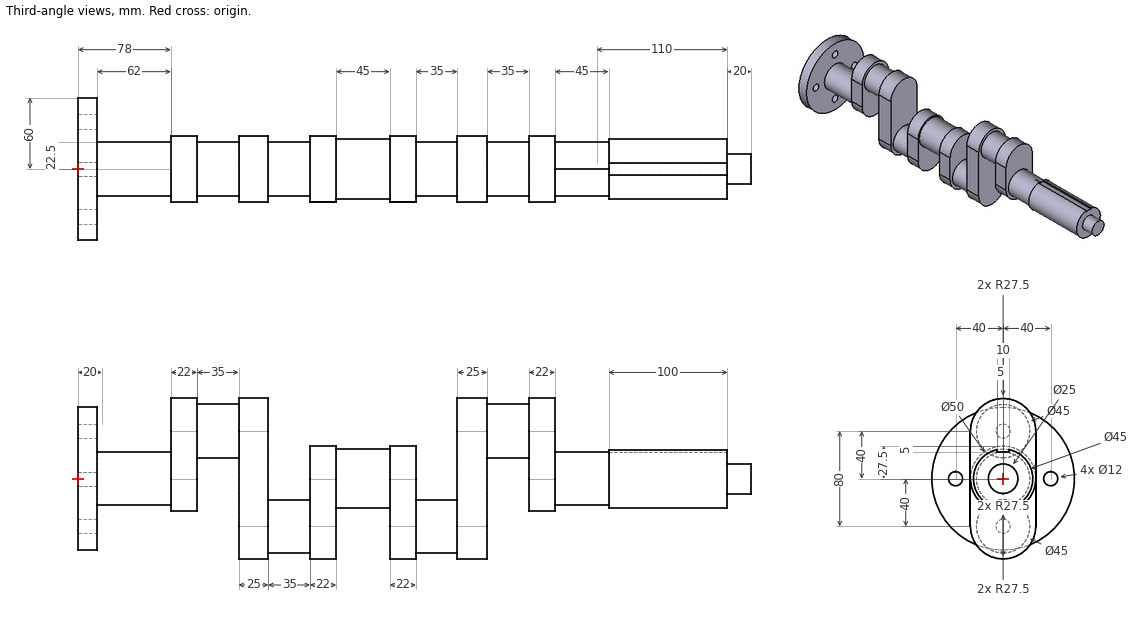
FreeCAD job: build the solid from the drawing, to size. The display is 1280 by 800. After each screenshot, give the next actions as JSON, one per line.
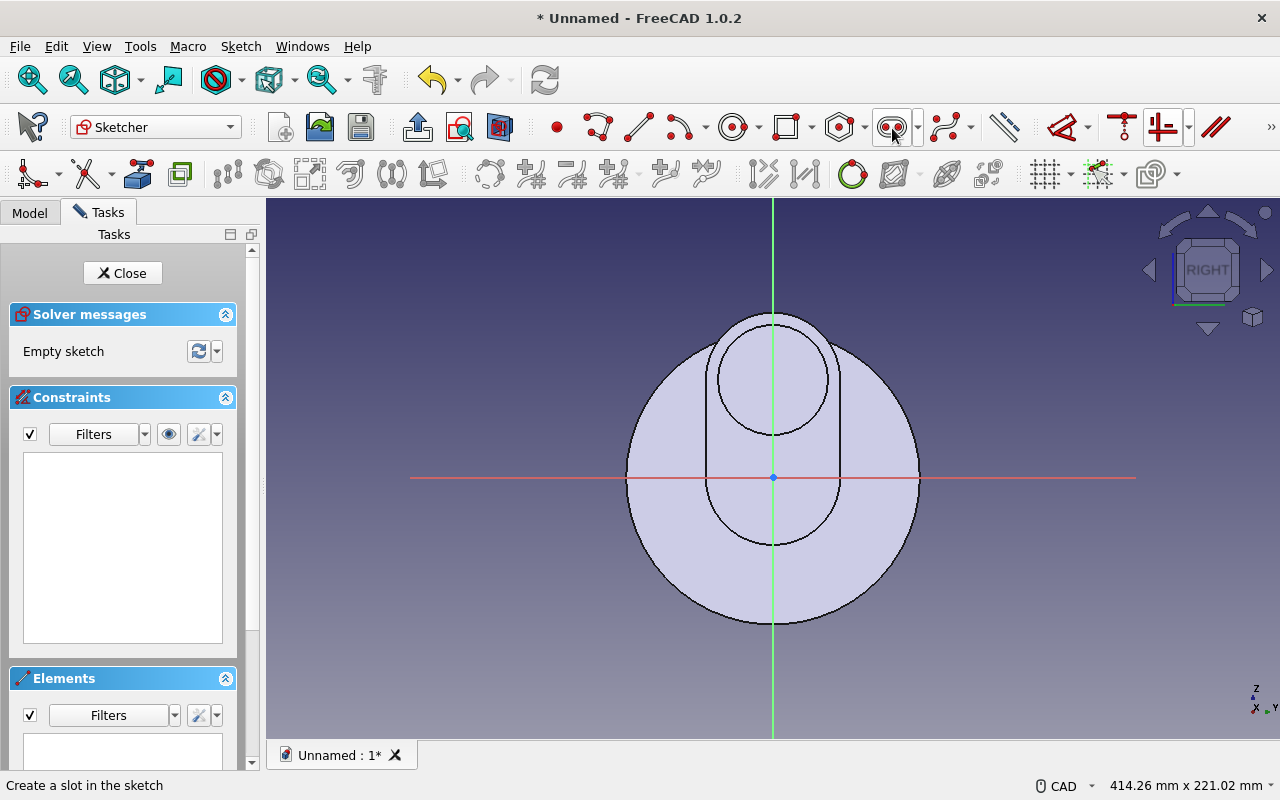
{"action": "left_click", "coordinate": [773, 576]}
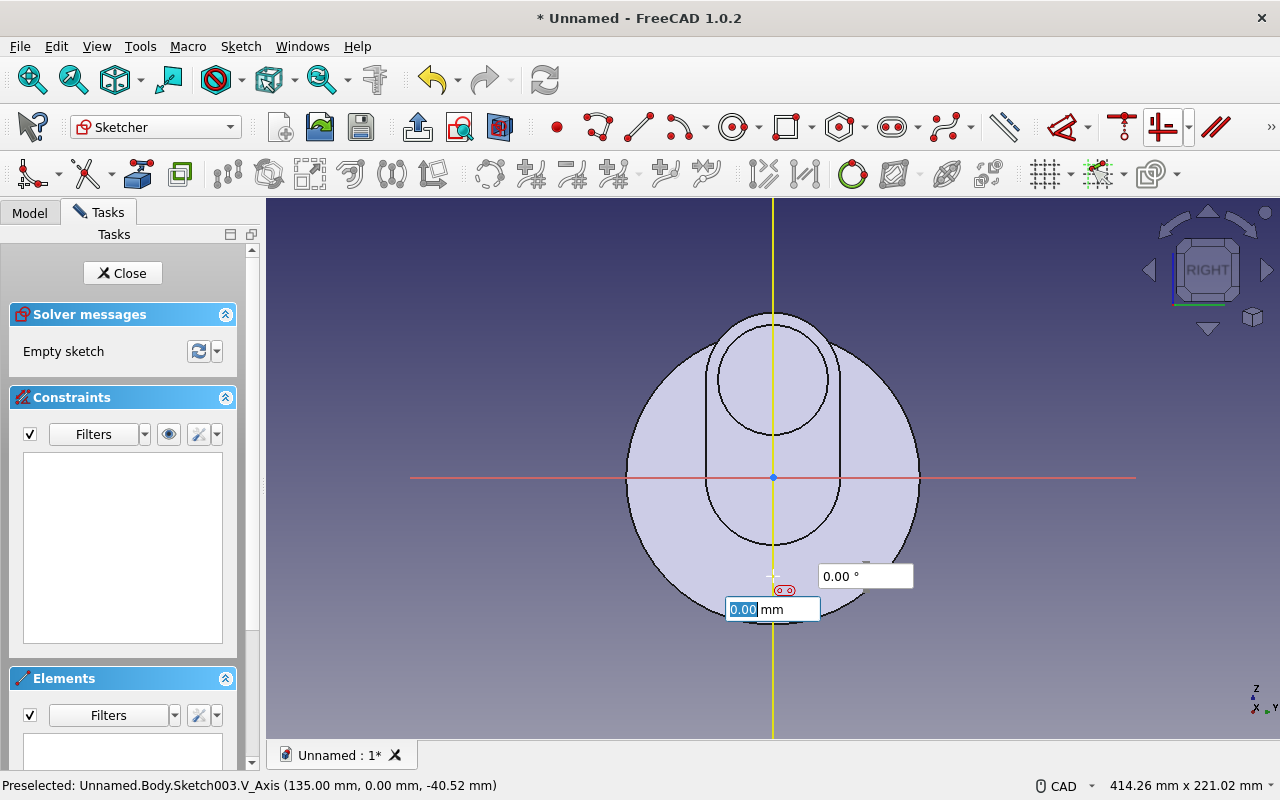
{"action": "left_click", "coordinate": [782, 380]}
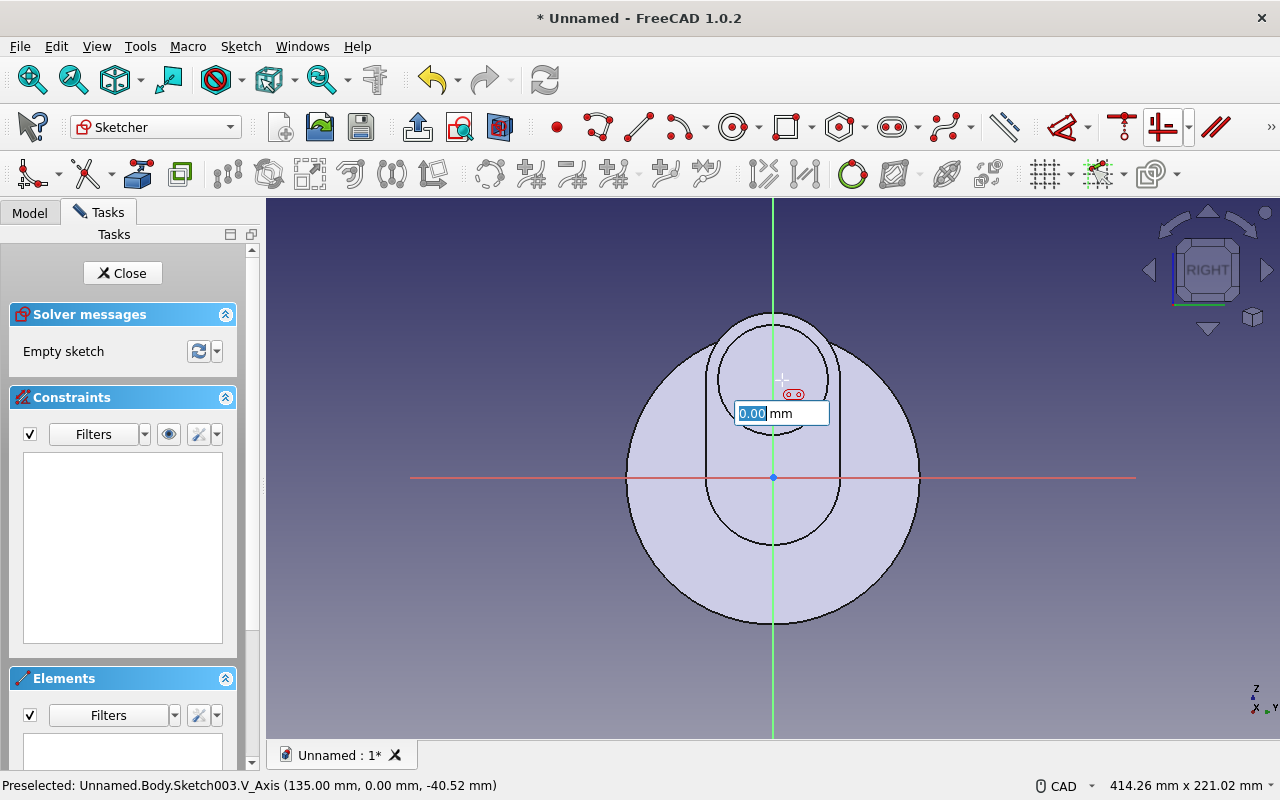
{"action": "left_click", "coordinate": [840, 507]}
{"action": "key", "text": "Escape"}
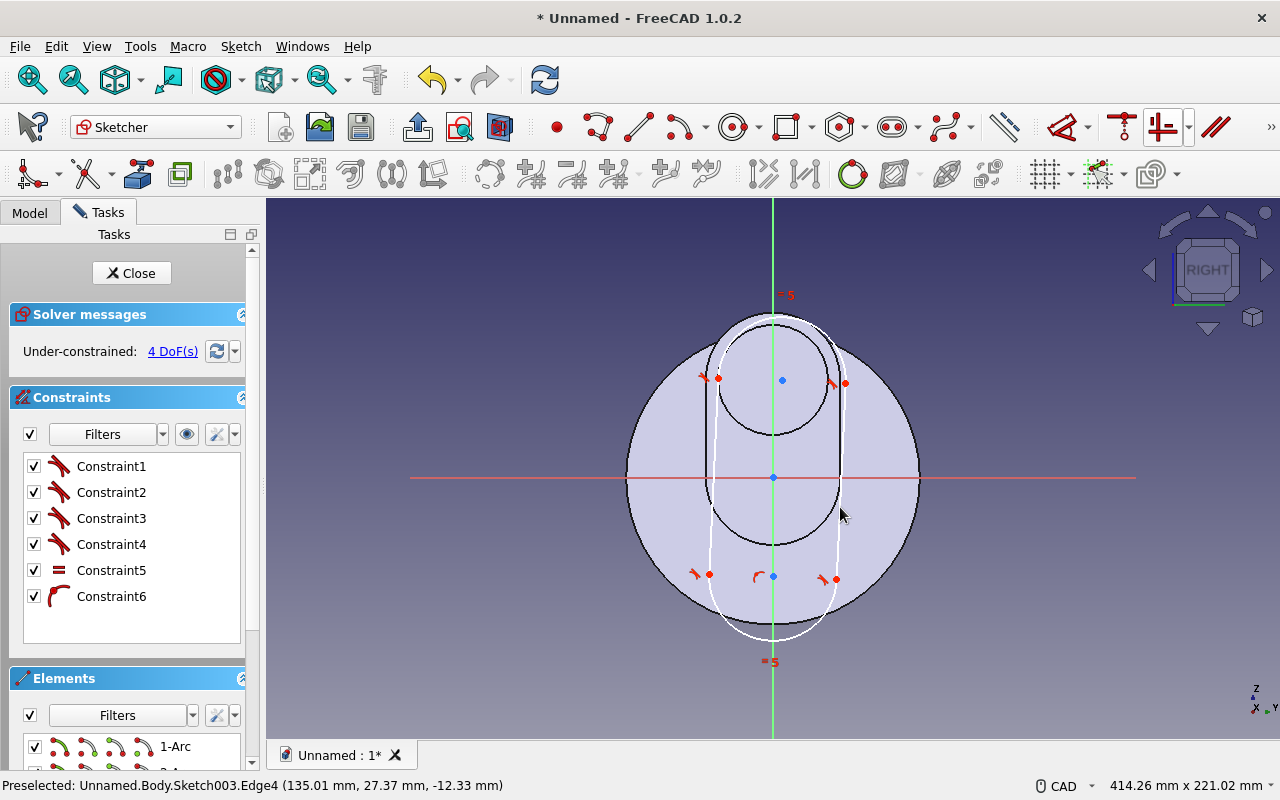
{"action": "left_click", "coordinate": [712, 515]}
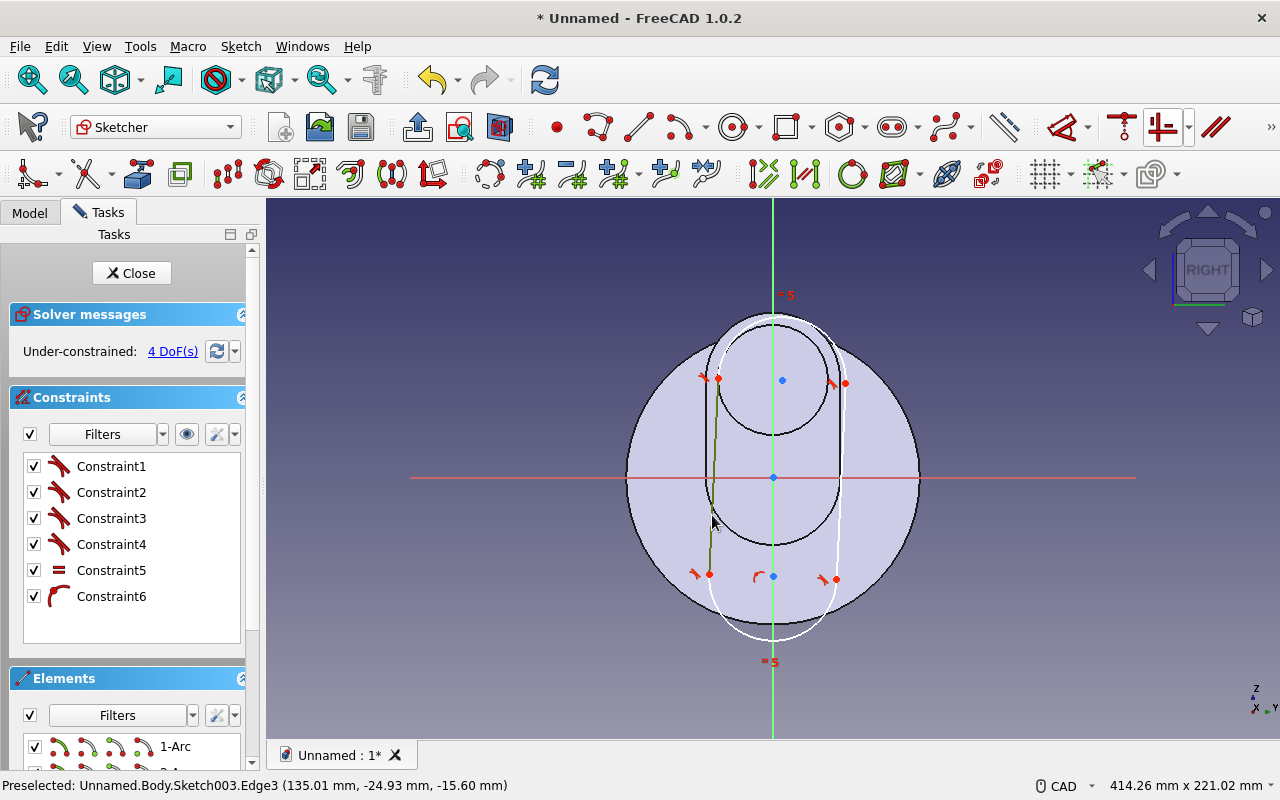
{"action": "left_click", "coordinate": [1188, 128]}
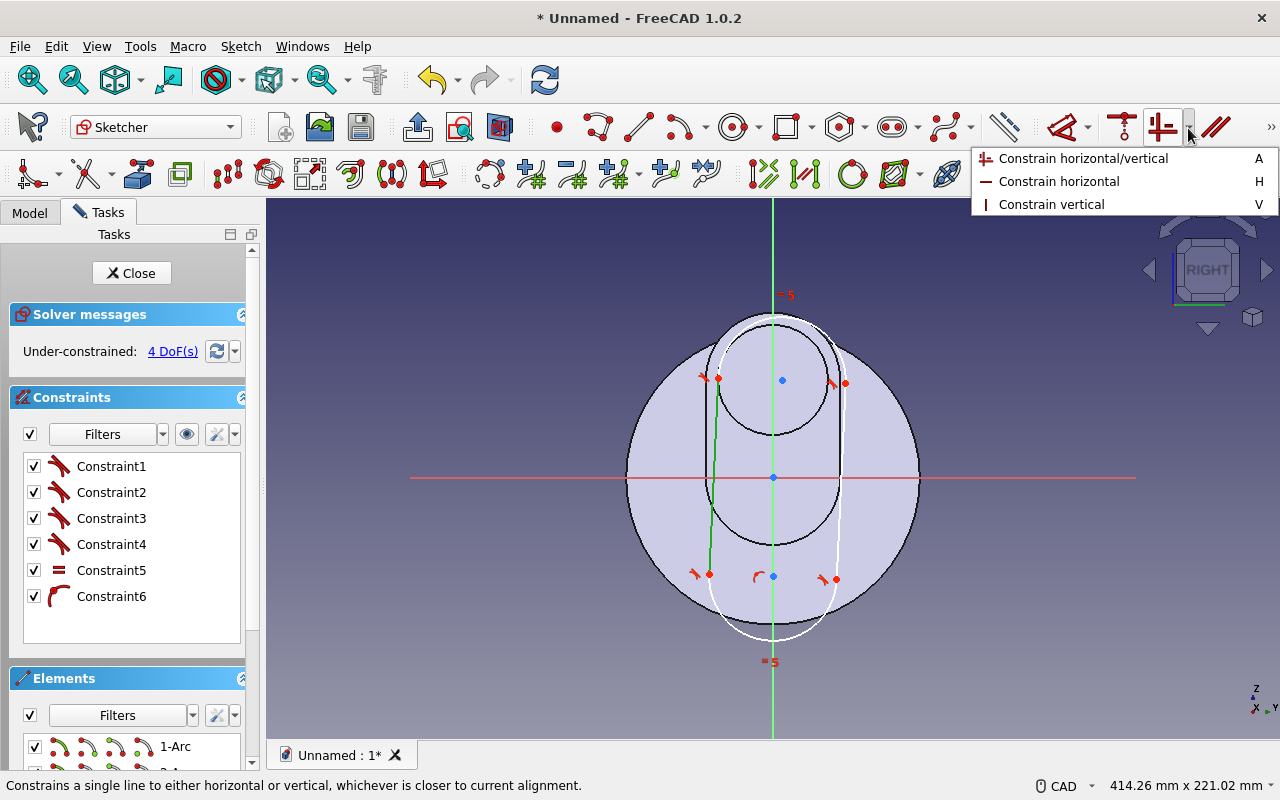
{"action": "left_click", "coordinate": [1125, 204]}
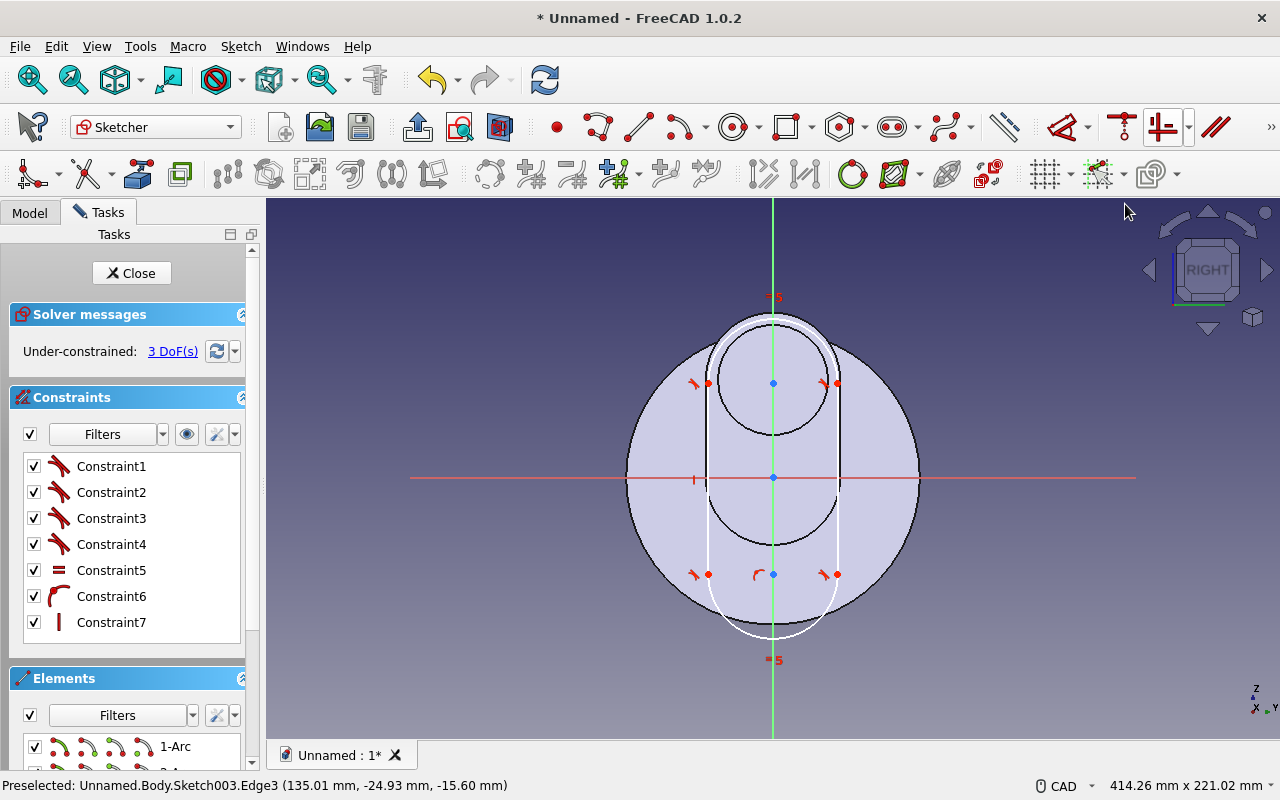
{"action": "left_click", "coordinate": [1062, 128]}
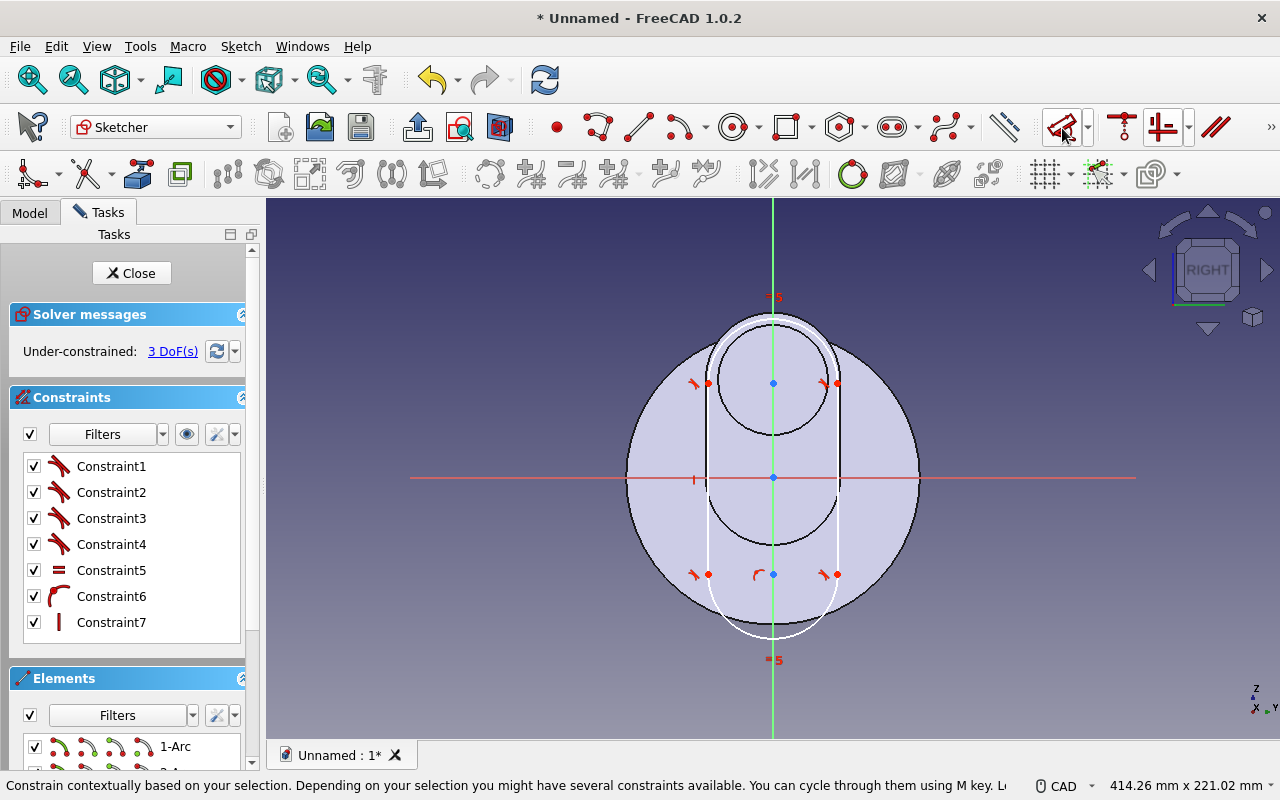
{"action": "left_click", "coordinate": [735, 626]}
{"action": "left_click", "coordinate": [716, 652]}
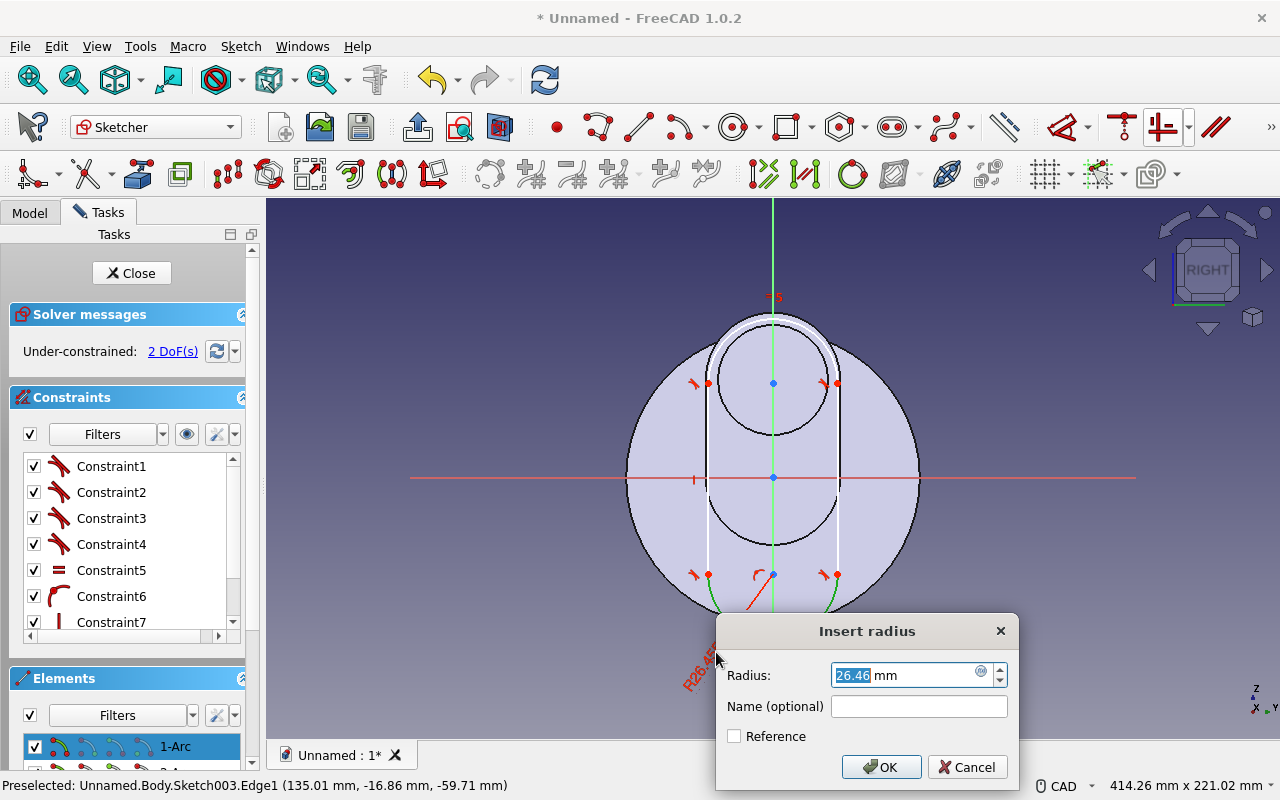
{"action": "type", "text": "27.5"}
{"action": "key", "text": "Return"}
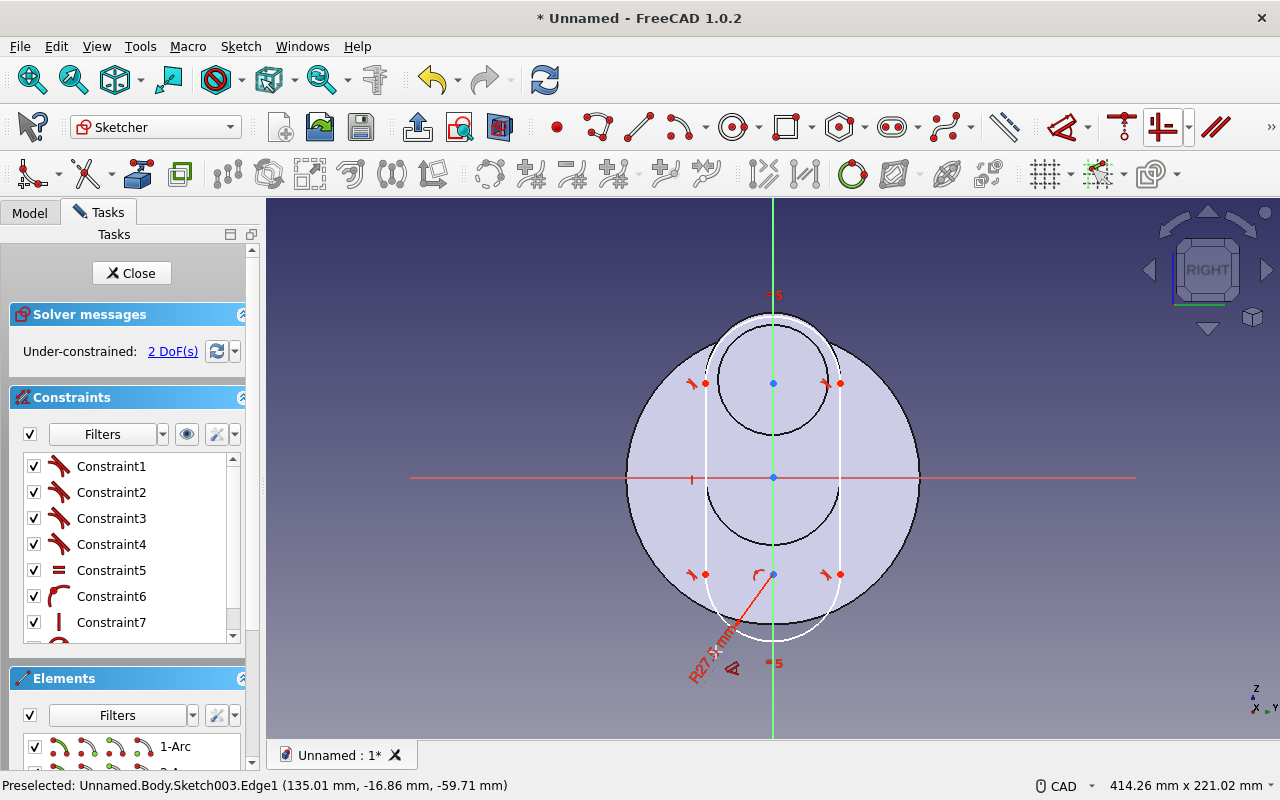
{"action": "left_click", "coordinate": [706, 517]}
{"action": "left_click", "coordinate": [672, 435]}